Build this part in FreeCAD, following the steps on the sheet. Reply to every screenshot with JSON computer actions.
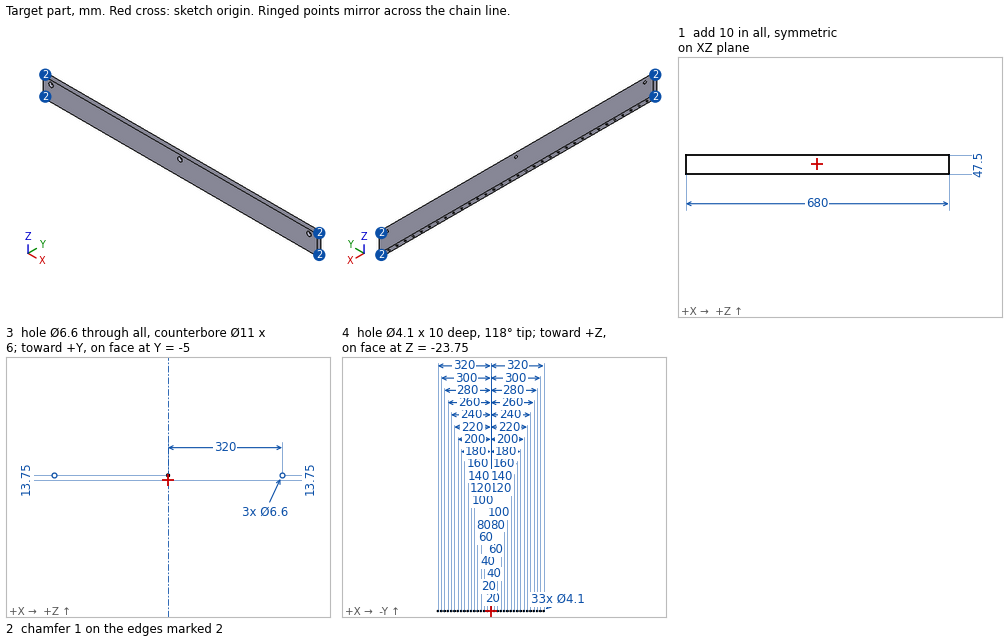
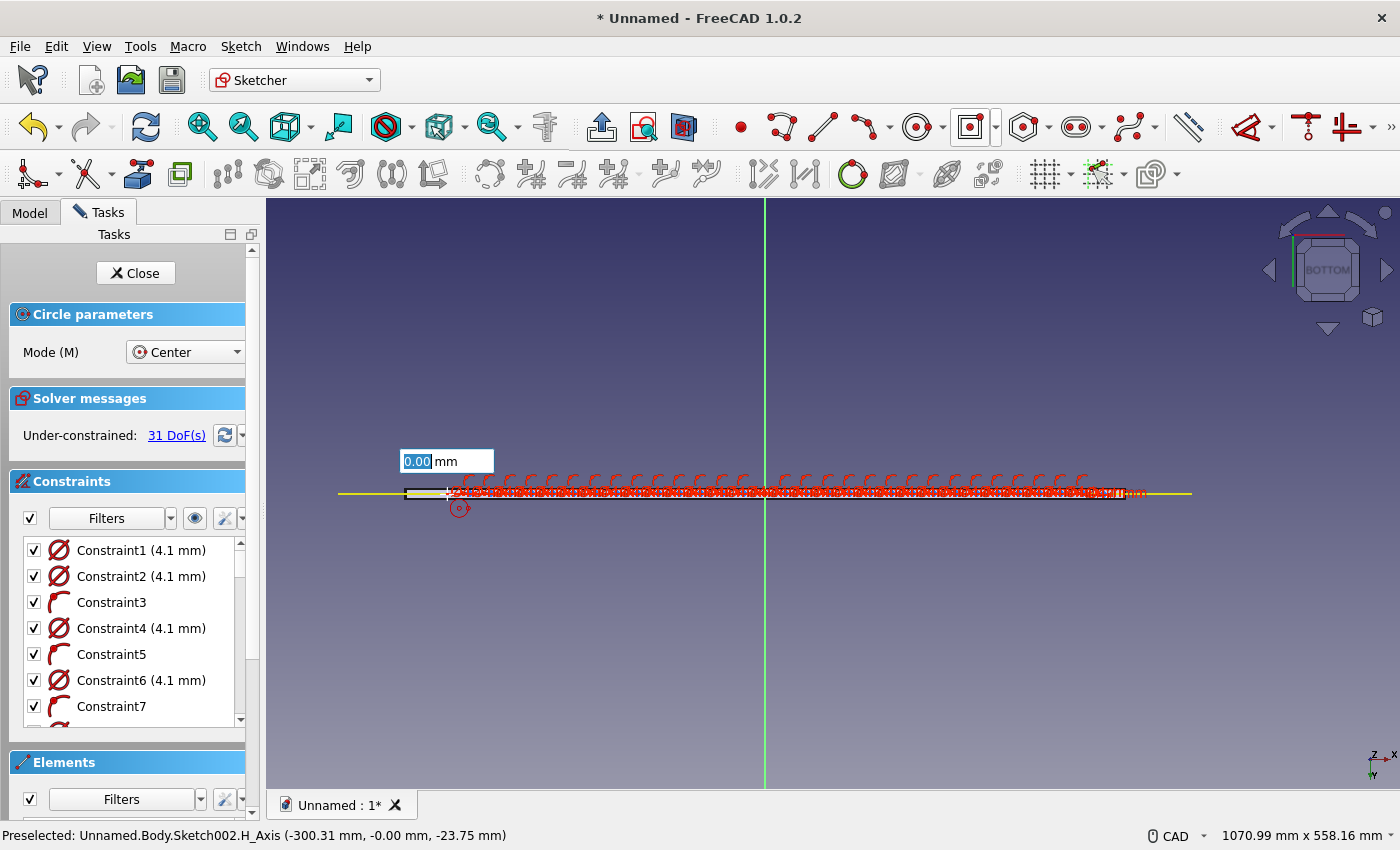
{"action": "scroll", "coordinate": [448, 492], "scroll_direction": "up", "scroll_amount": 11}
{"action": "mouse_move", "coordinate": [447, 486]}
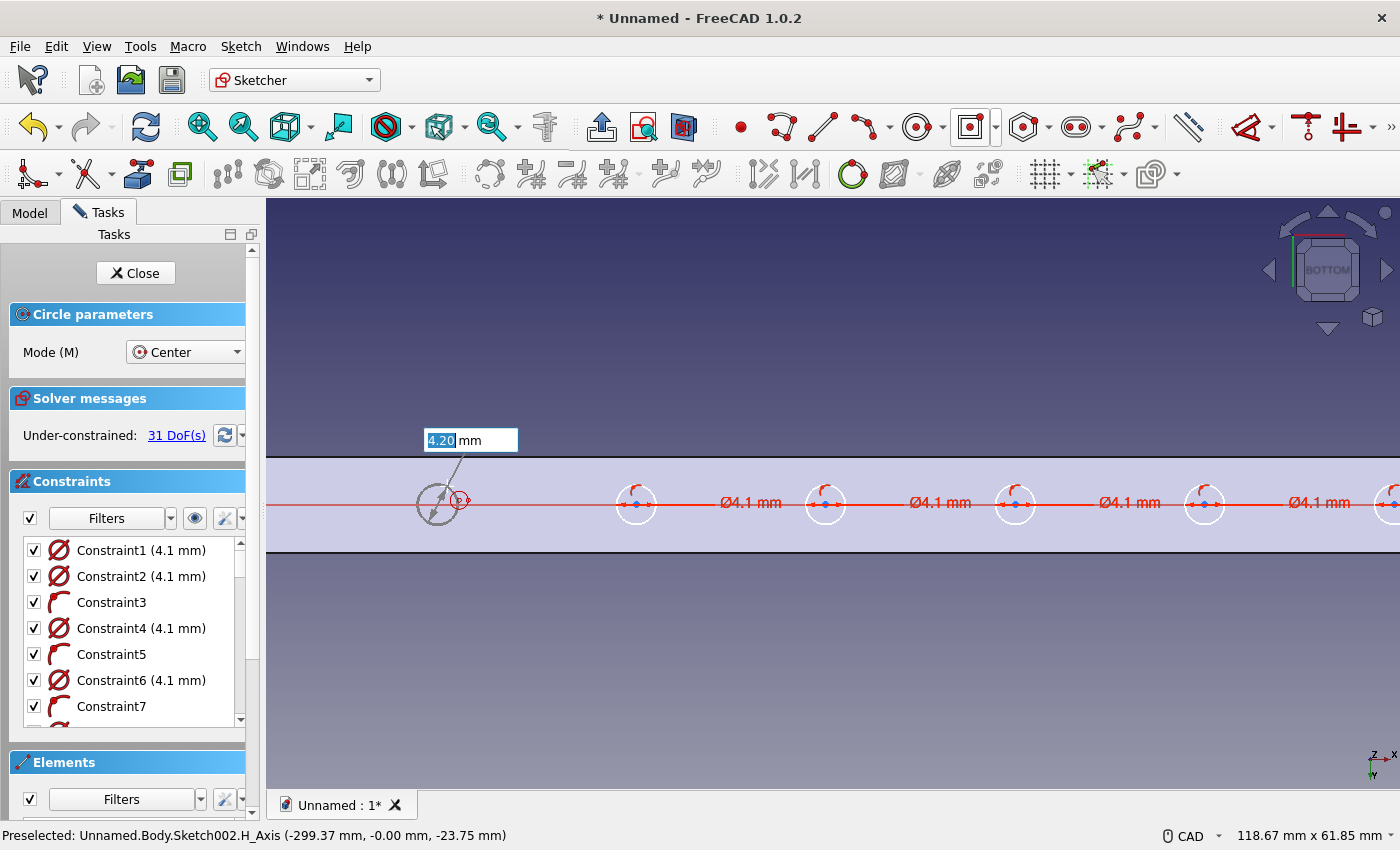
{"action": "type", "text": "4.1"}
{"action": "key", "text": "Return"}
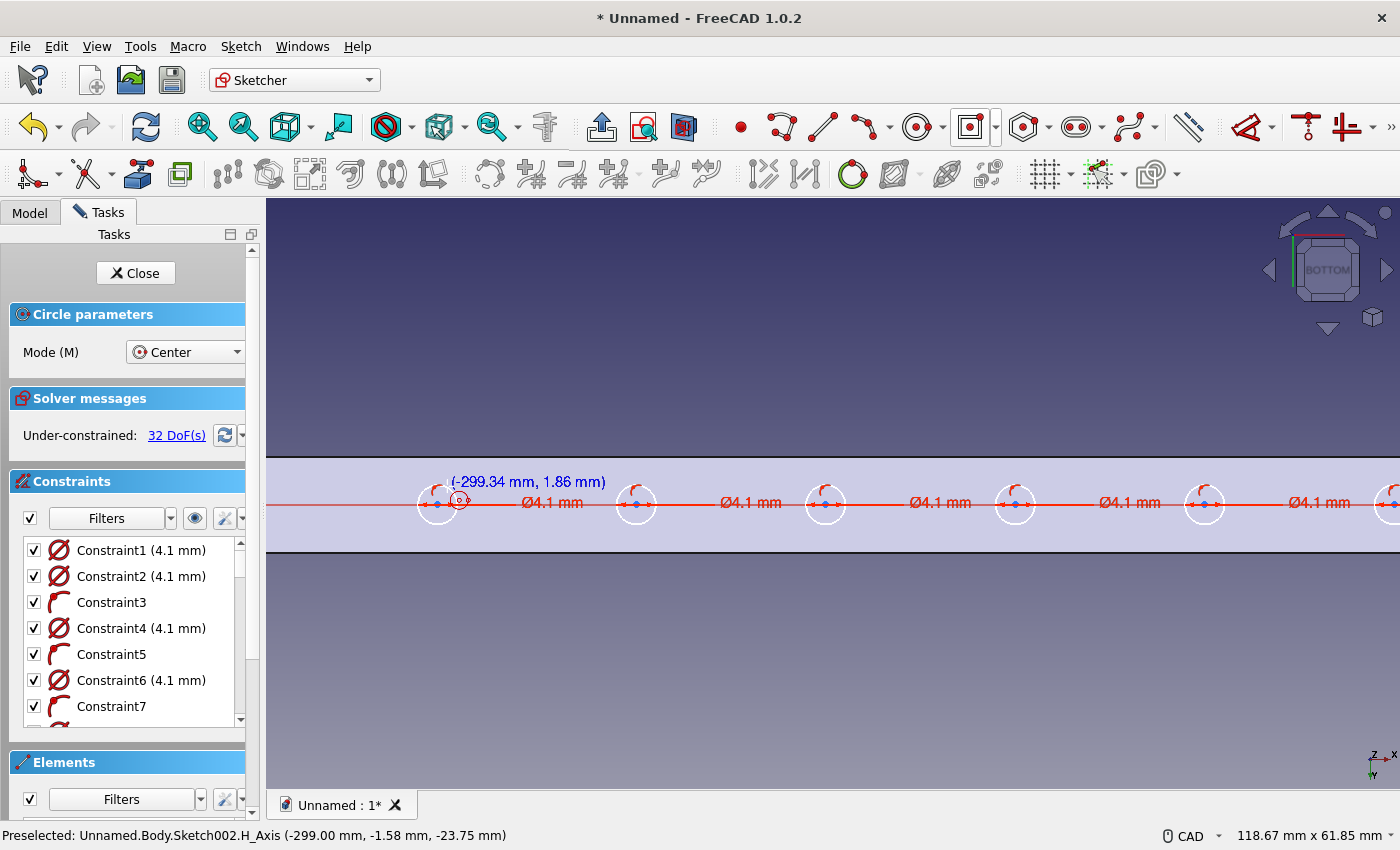
{"action": "scroll", "coordinate": [448, 492], "scroll_direction": "down", "scroll_amount": 11}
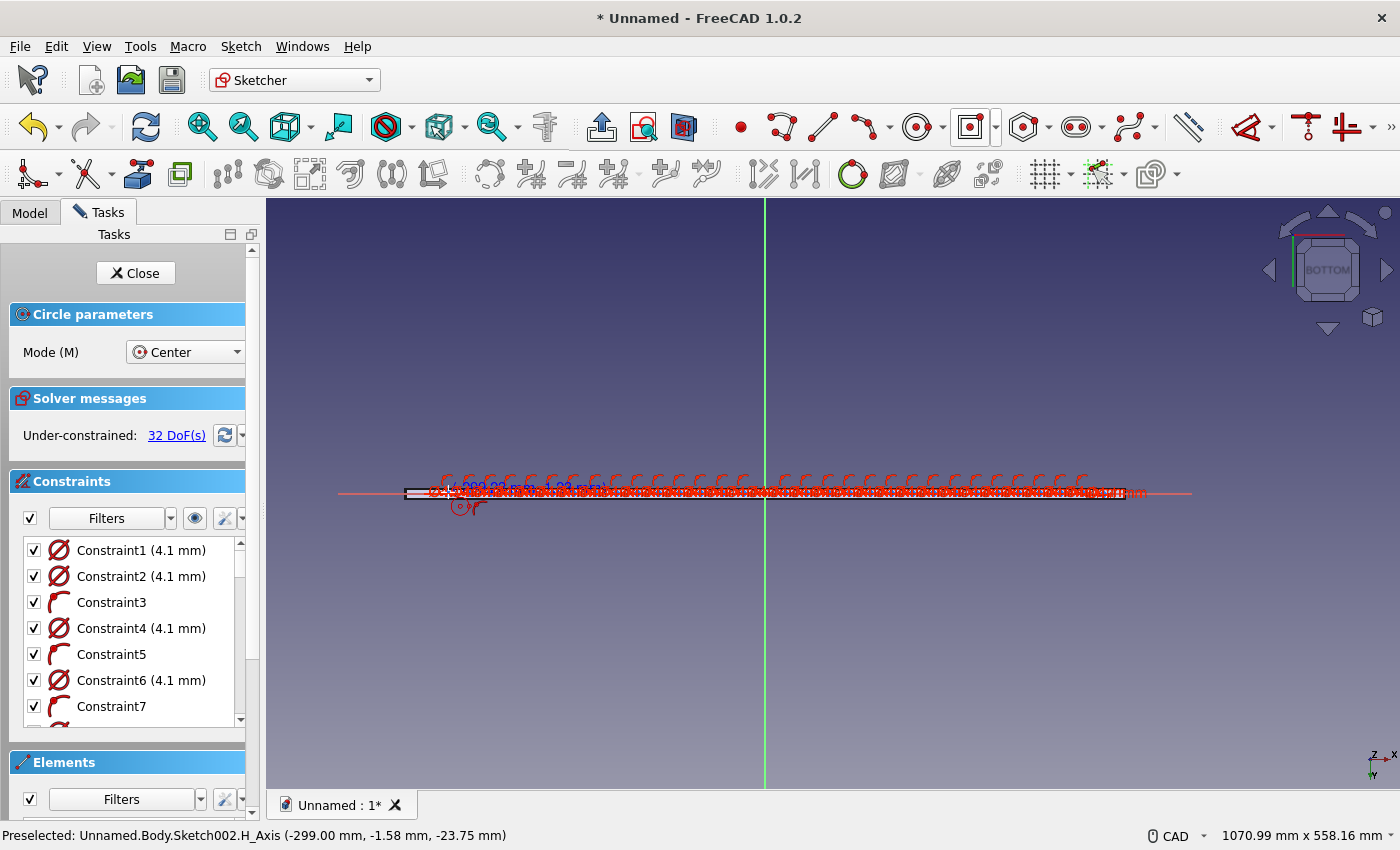
{"action": "scroll", "coordinate": [426, 494], "scroll_direction": "up", "scroll_amount": 12}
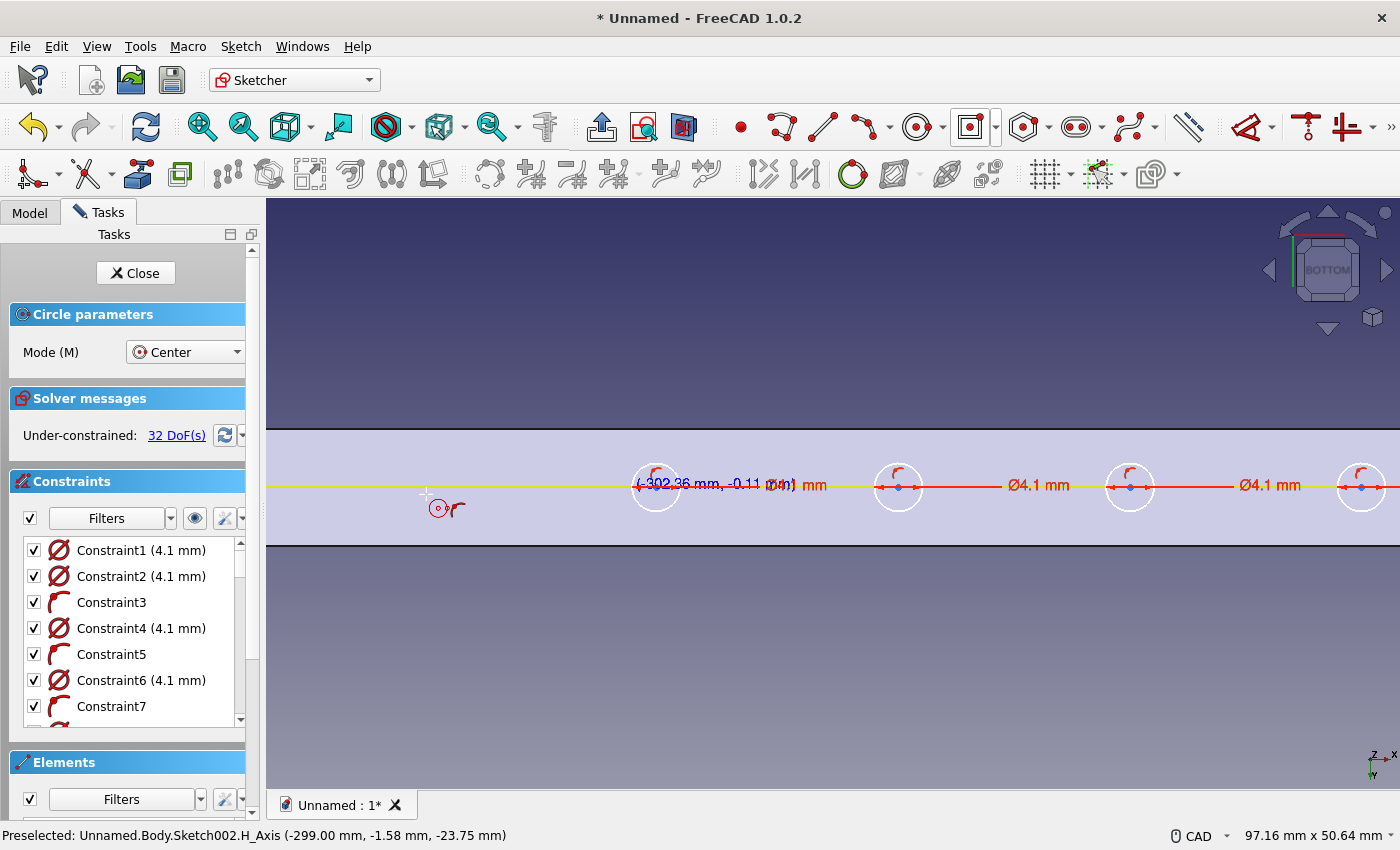
{"action": "scroll", "coordinate": [426, 494], "scroll_direction": "down", "scroll_amount": 12}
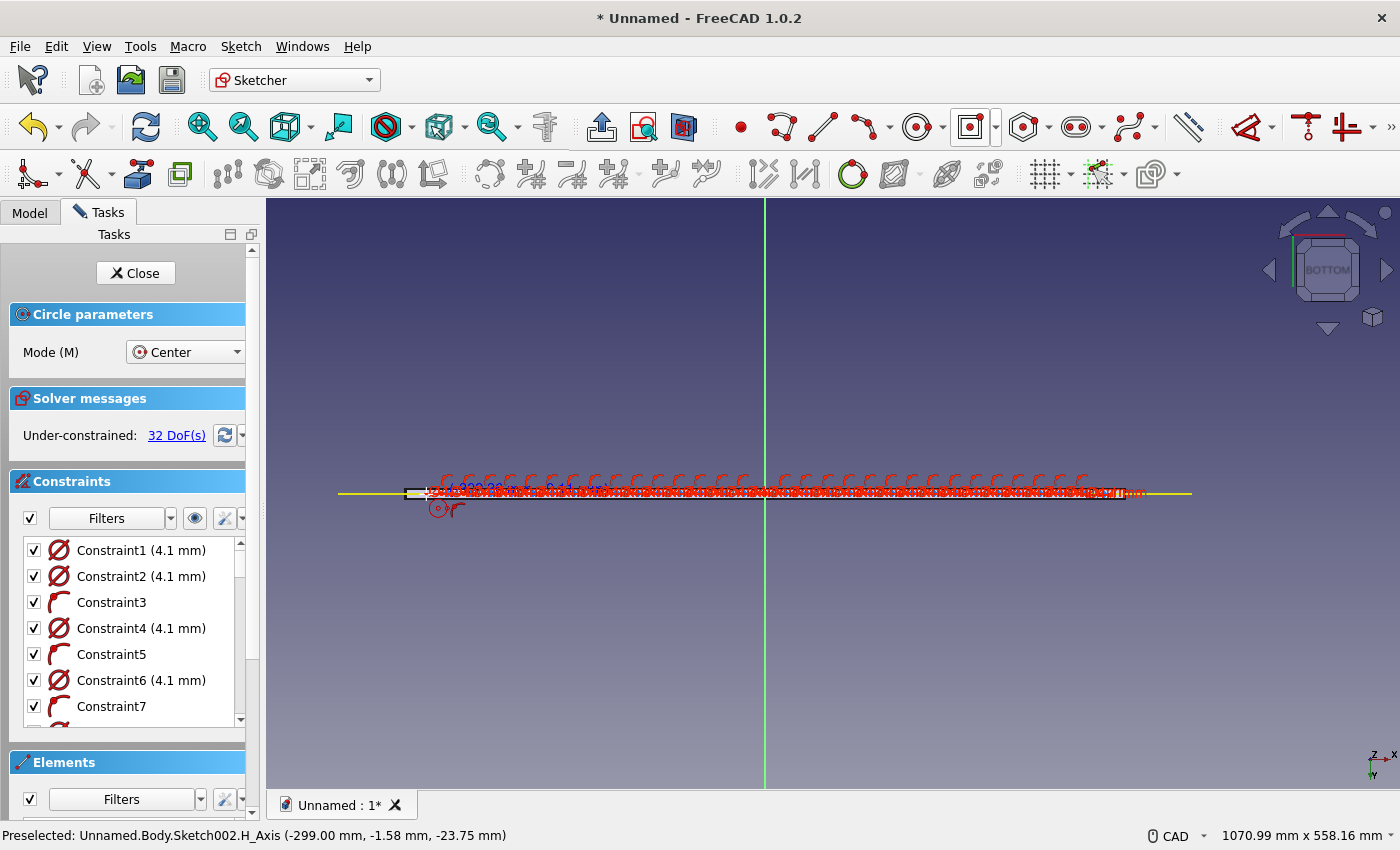
{"action": "left_click", "coordinate": [426, 494]}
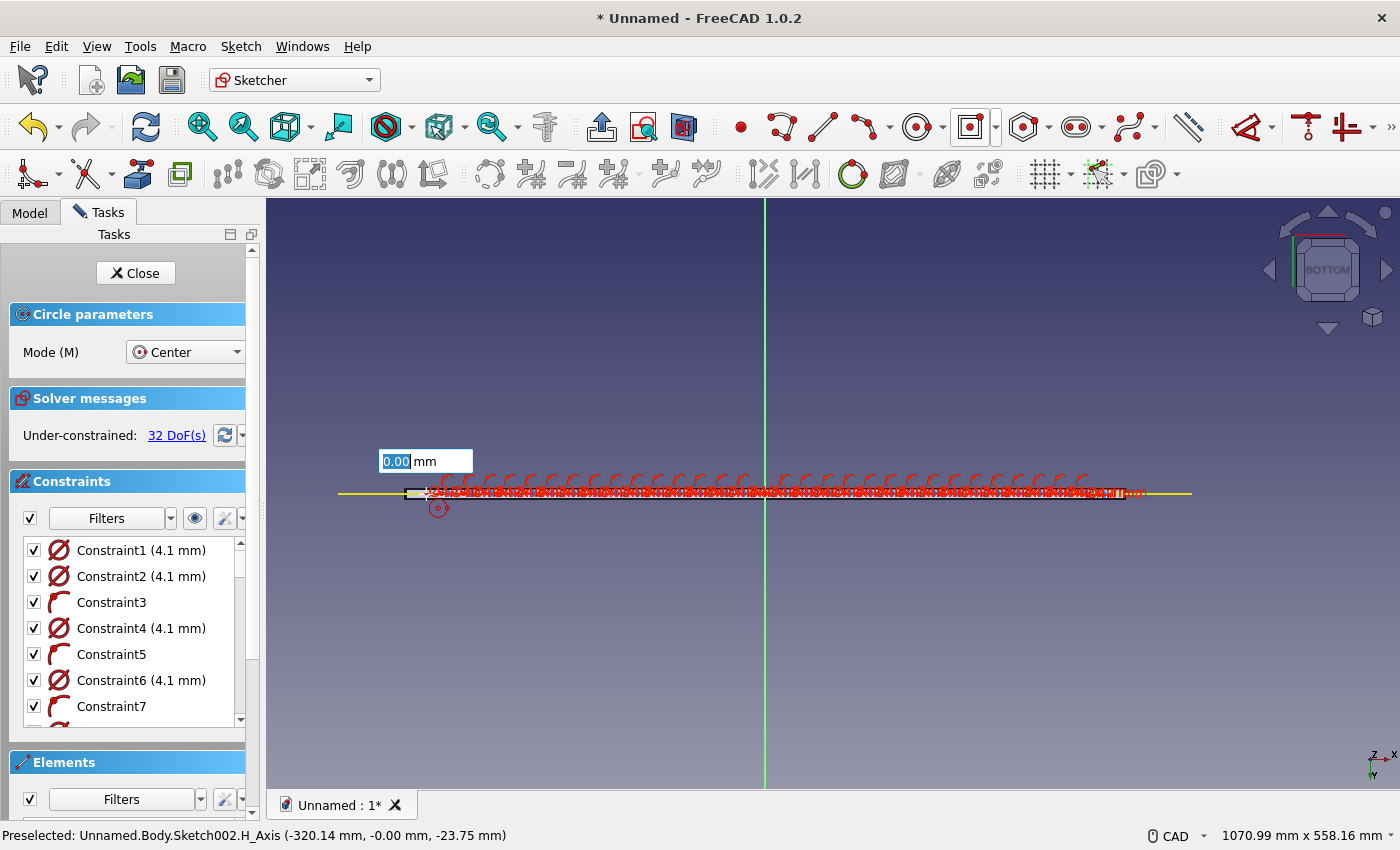
{"action": "scroll", "coordinate": [427, 492], "scroll_direction": "up", "scroll_amount": 11}
{"action": "mouse_move", "coordinate": [425, 486]}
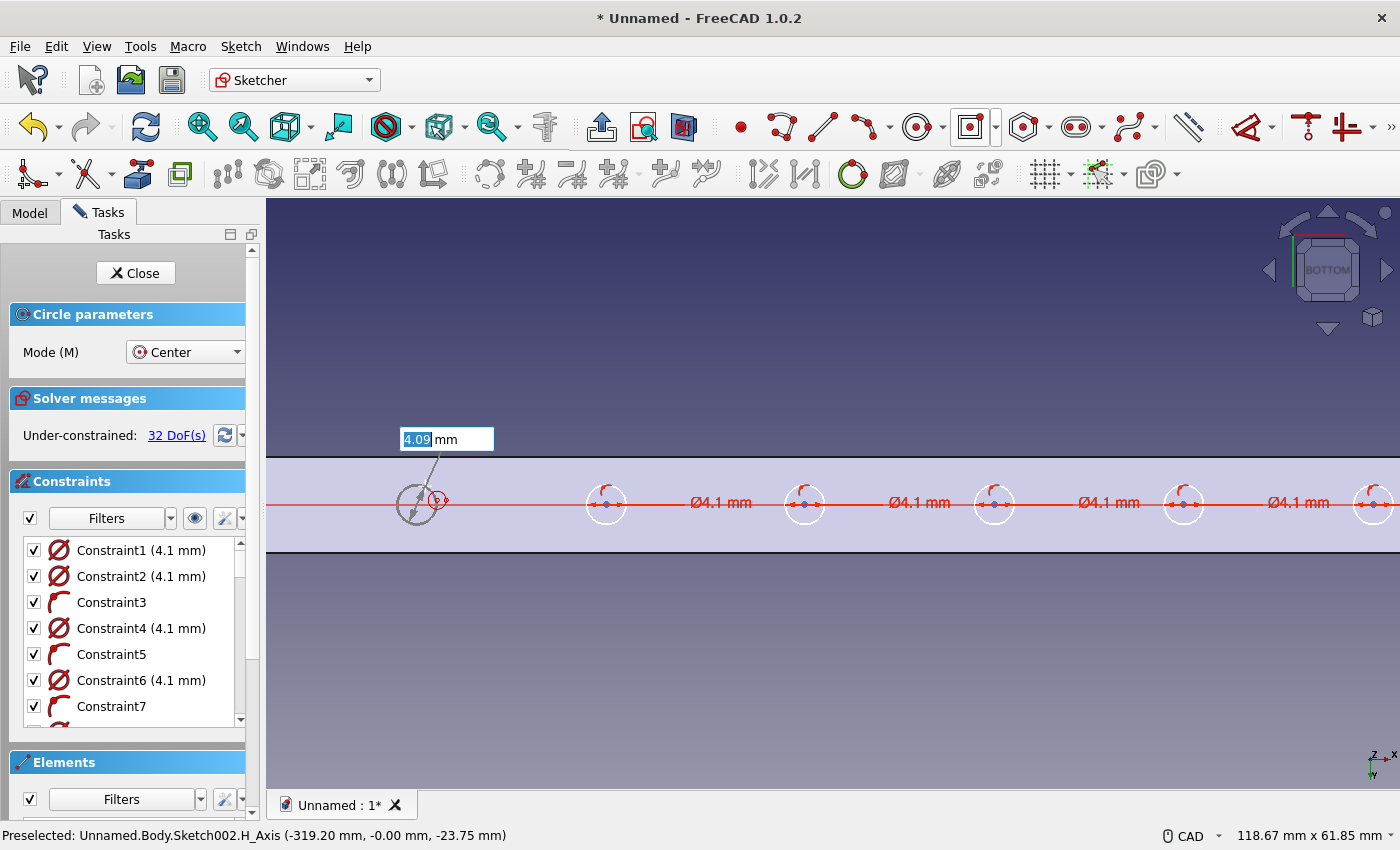
{"action": "type", "text": "4.1"}
{"action": "key", "text": "Return"}
{"action": "key", "text": "Escape"}